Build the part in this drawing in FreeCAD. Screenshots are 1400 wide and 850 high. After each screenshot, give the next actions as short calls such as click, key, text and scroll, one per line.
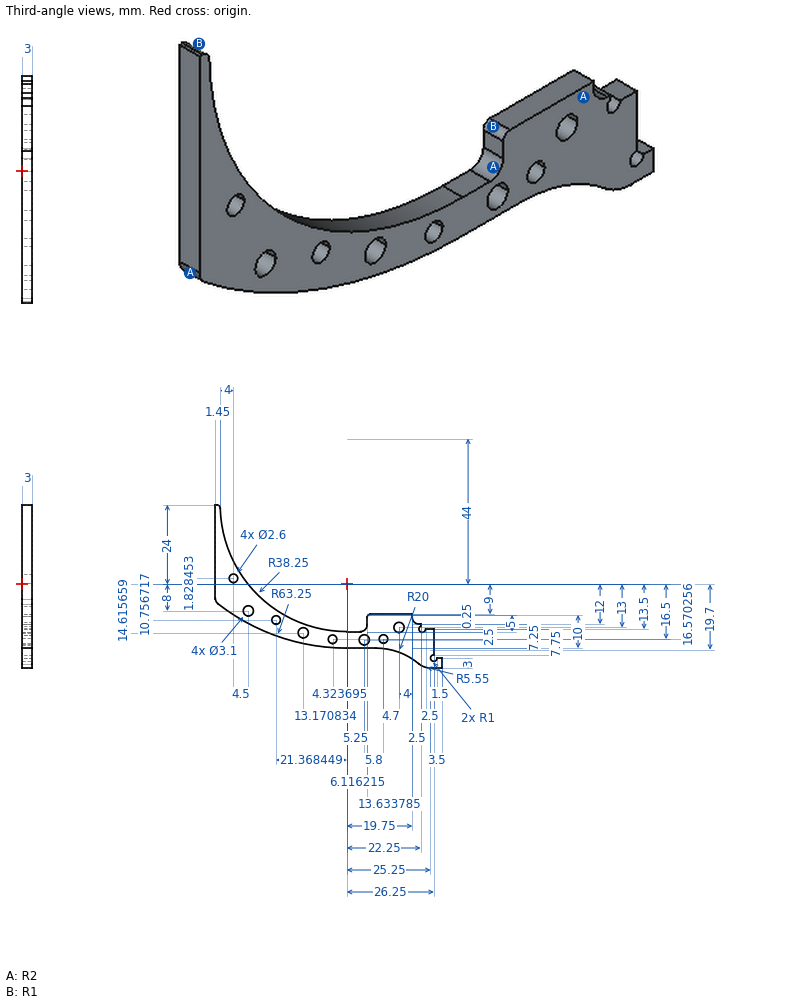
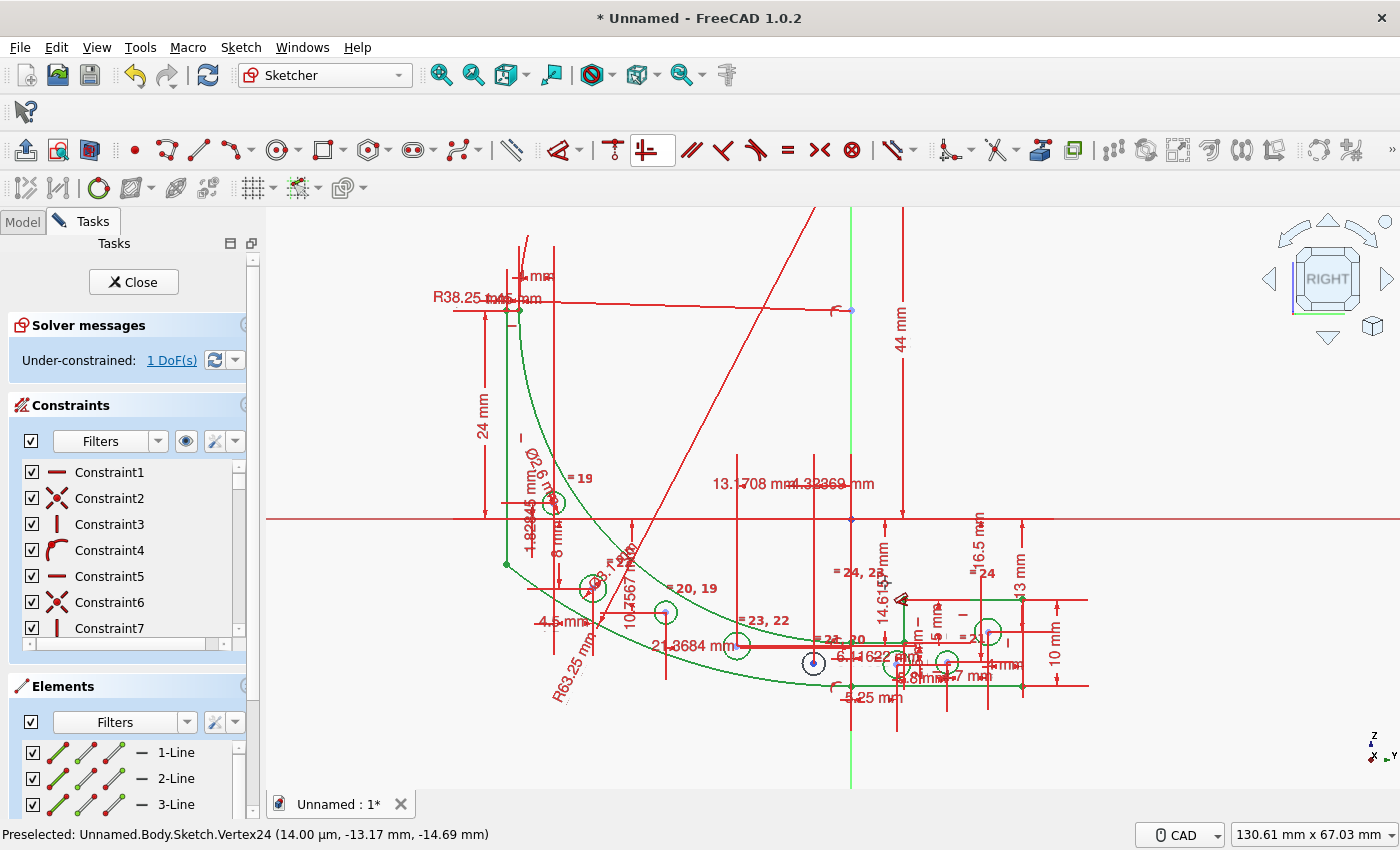
click(814, 664)
click(885, 558)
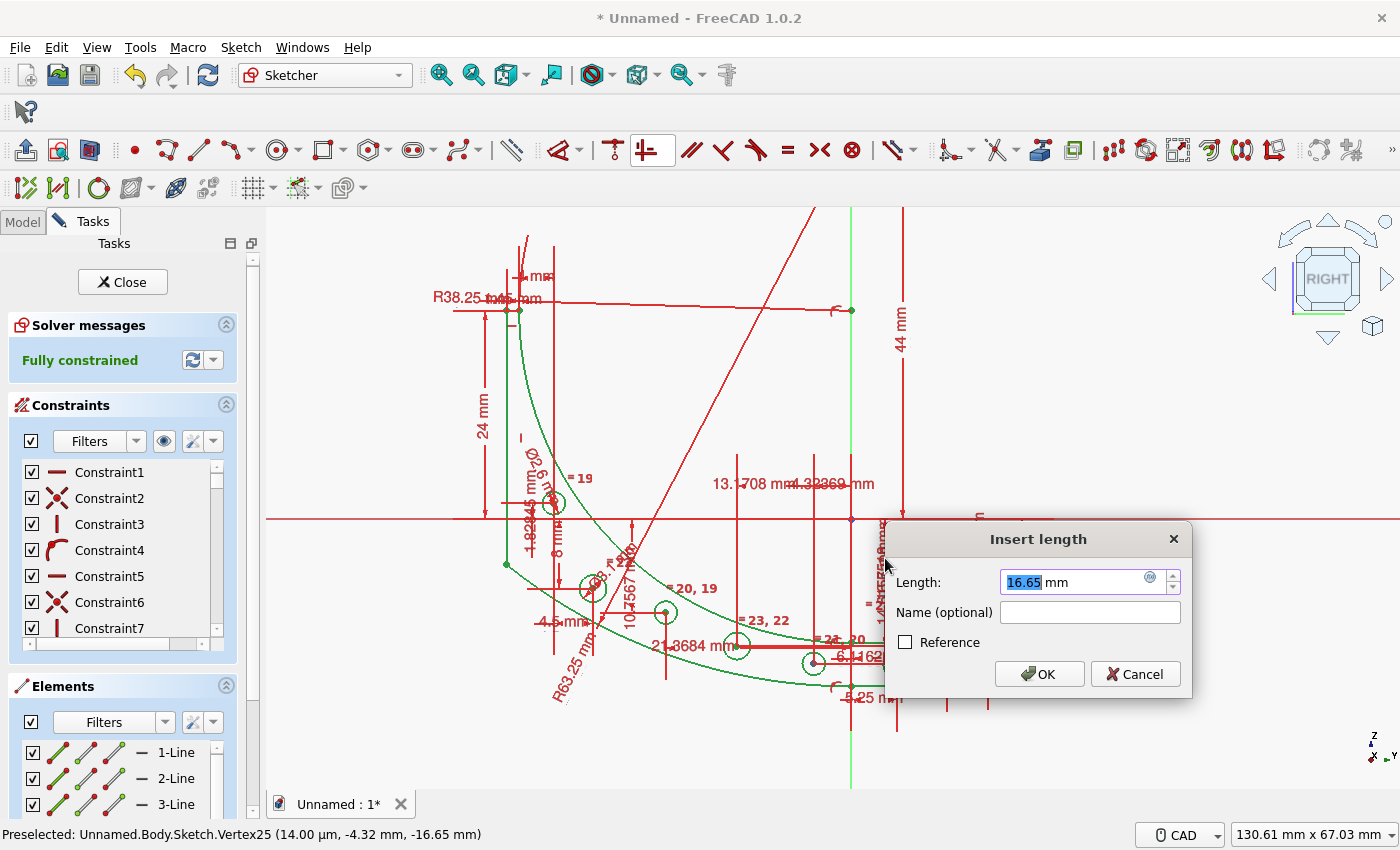
text(16.570256)
key(Return)
key(Escape)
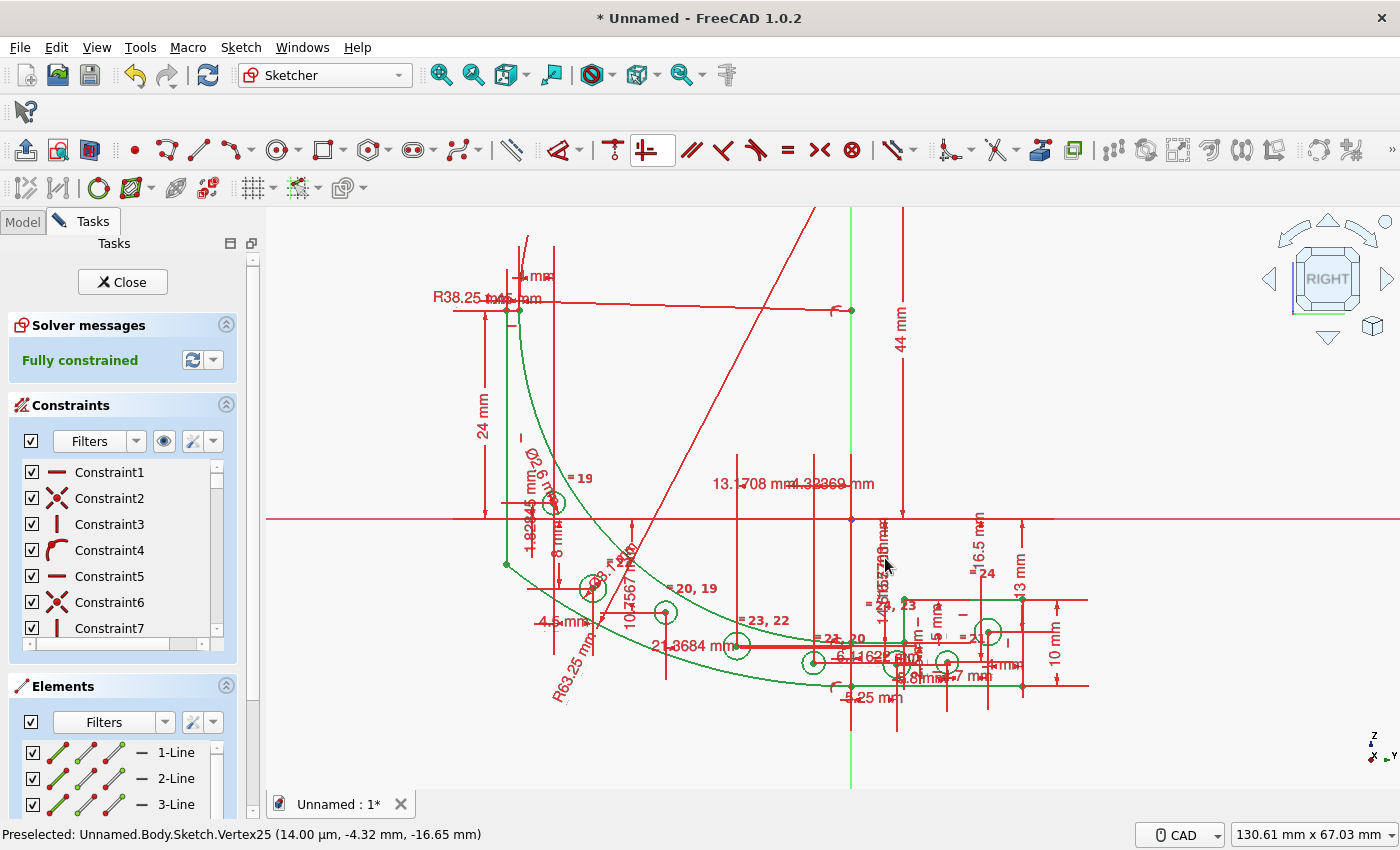
click(123, 282)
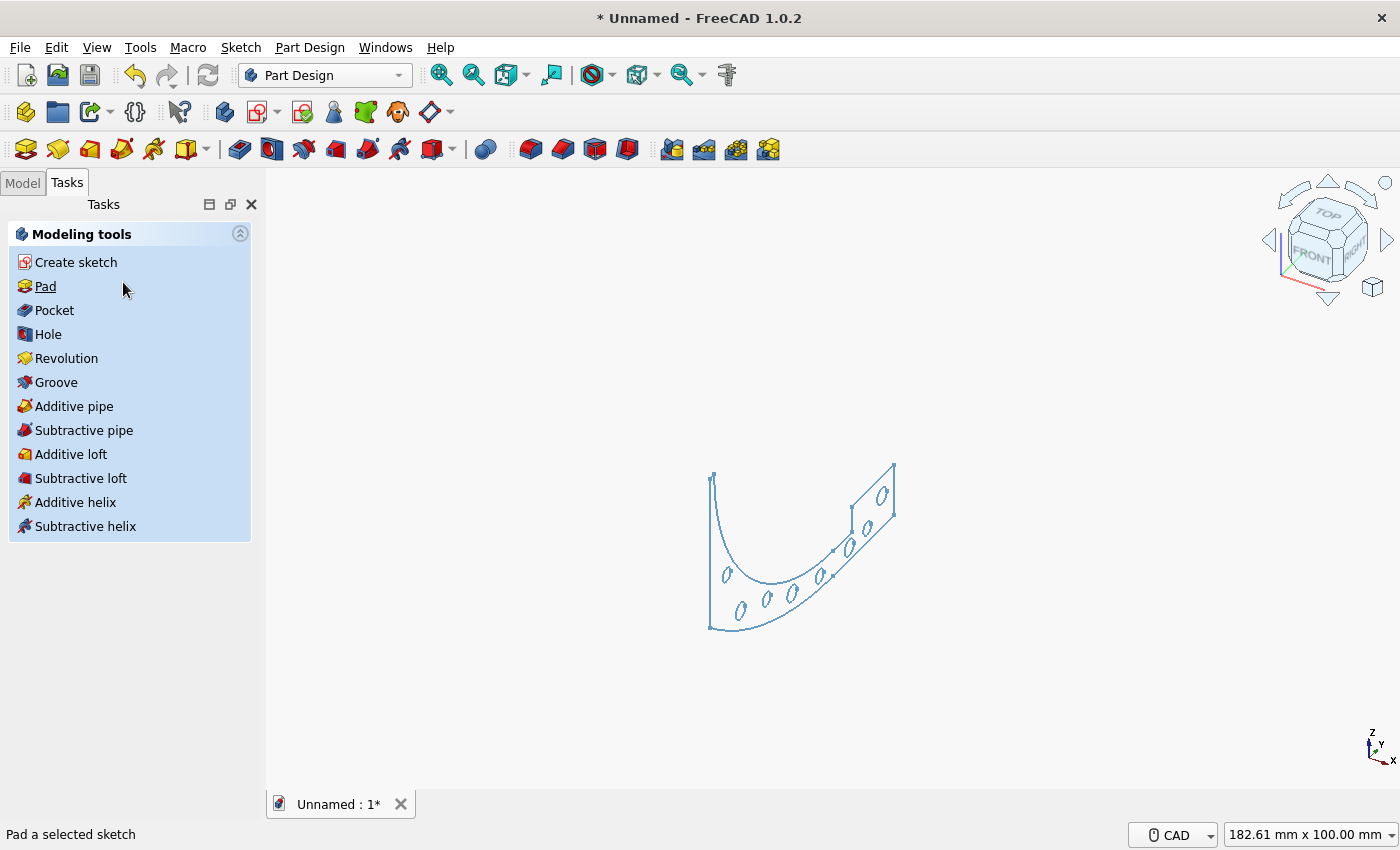
click(26, 150)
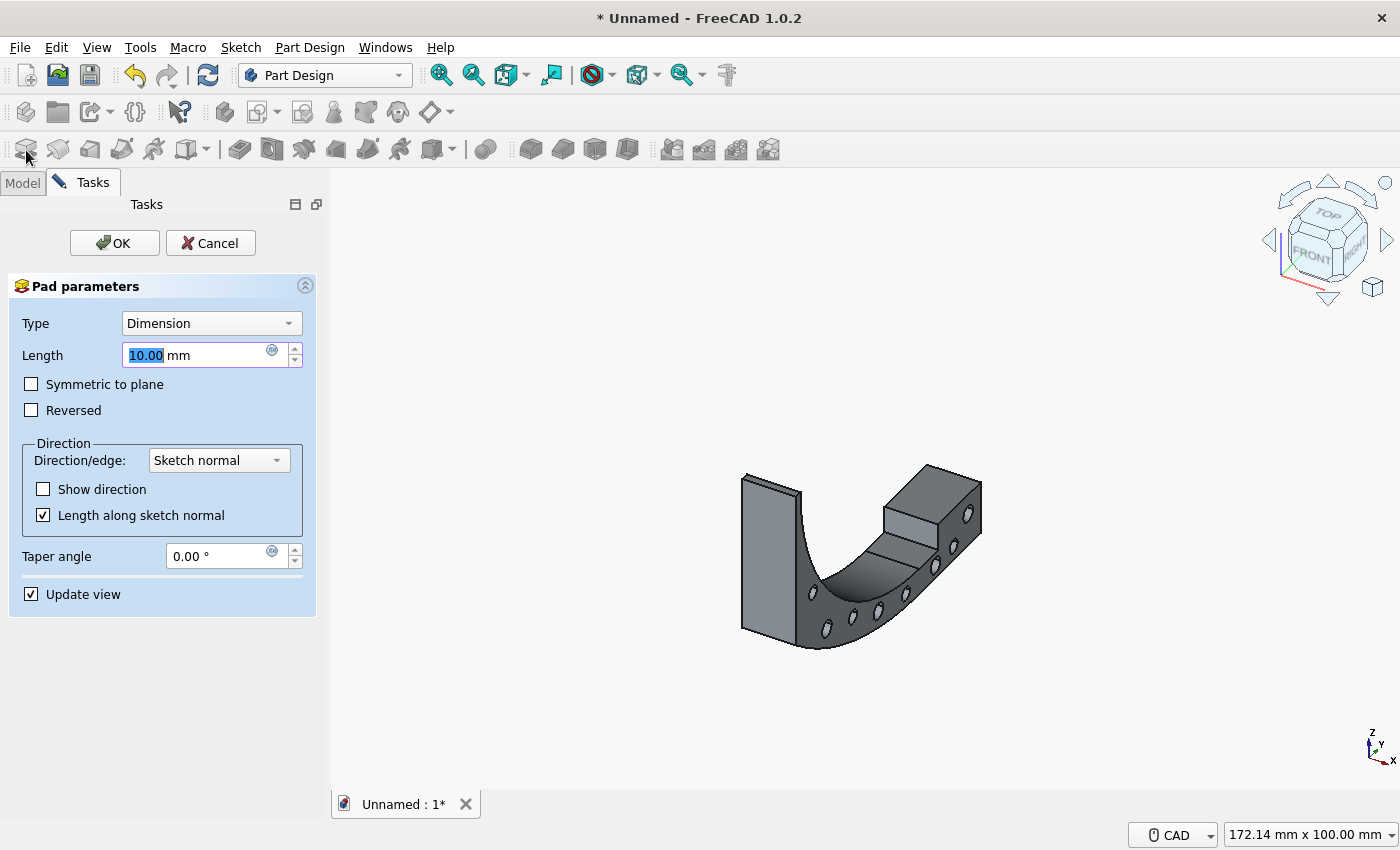
text(3)
key(Tab)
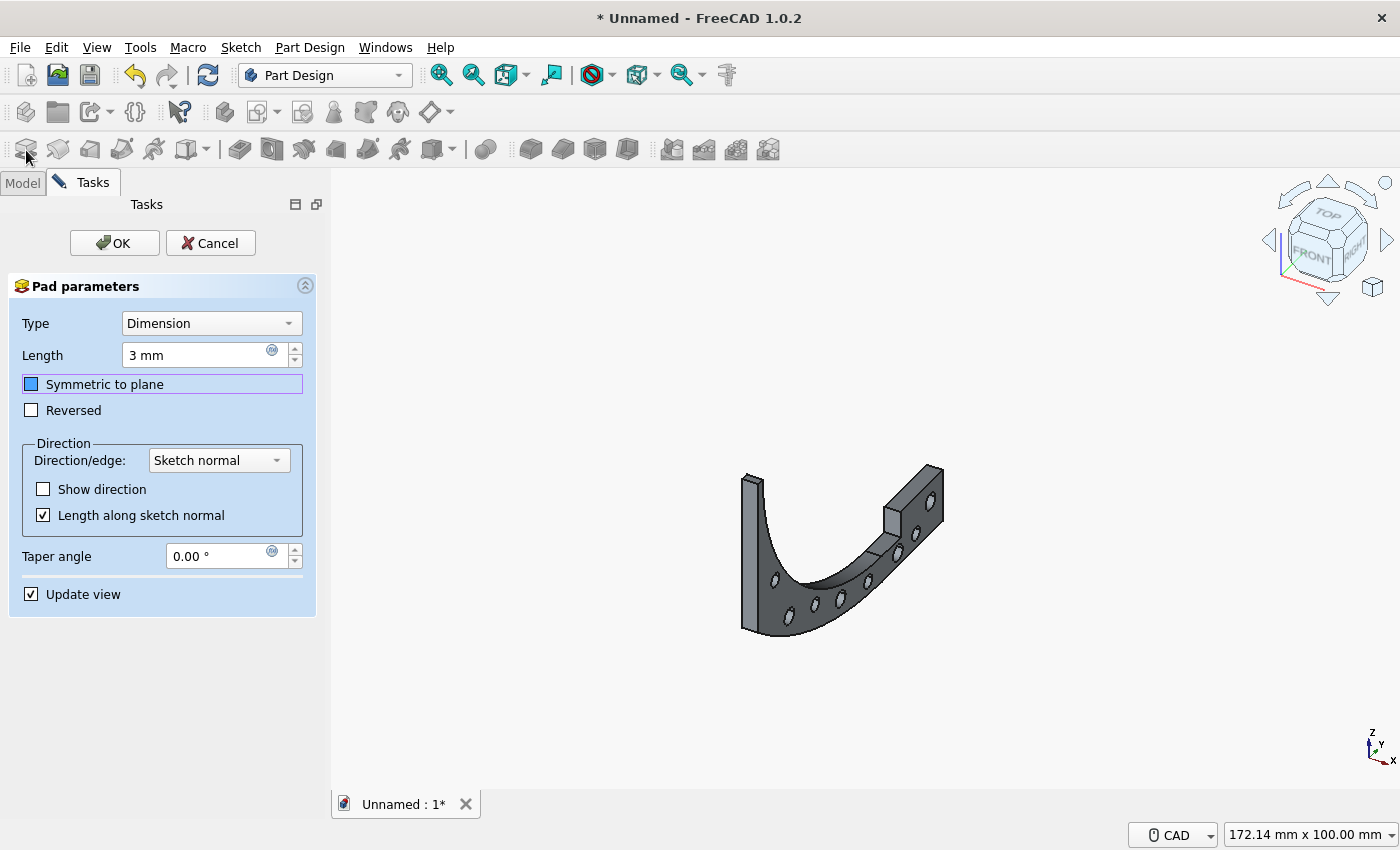
click(115, 243)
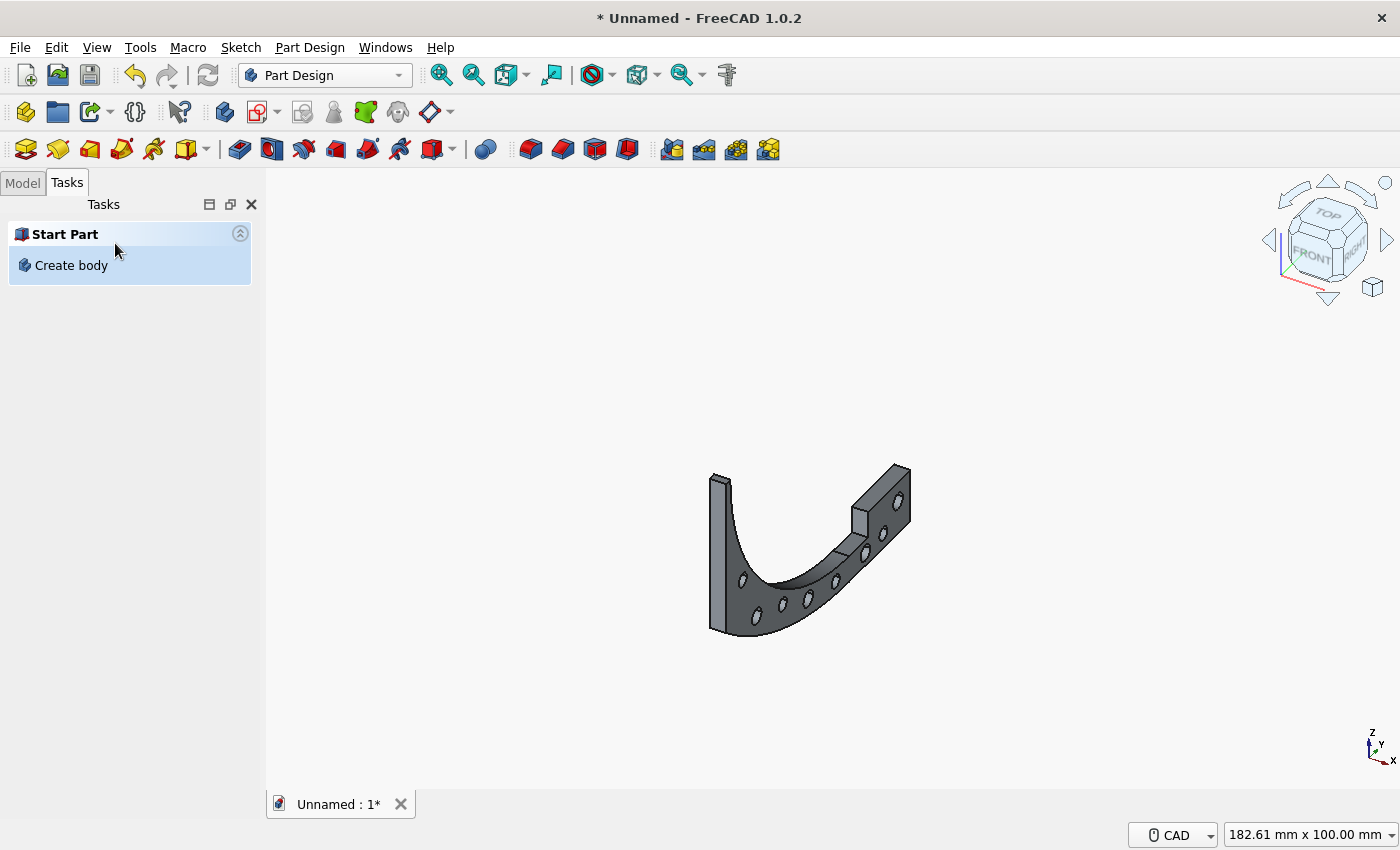
click(739, 612)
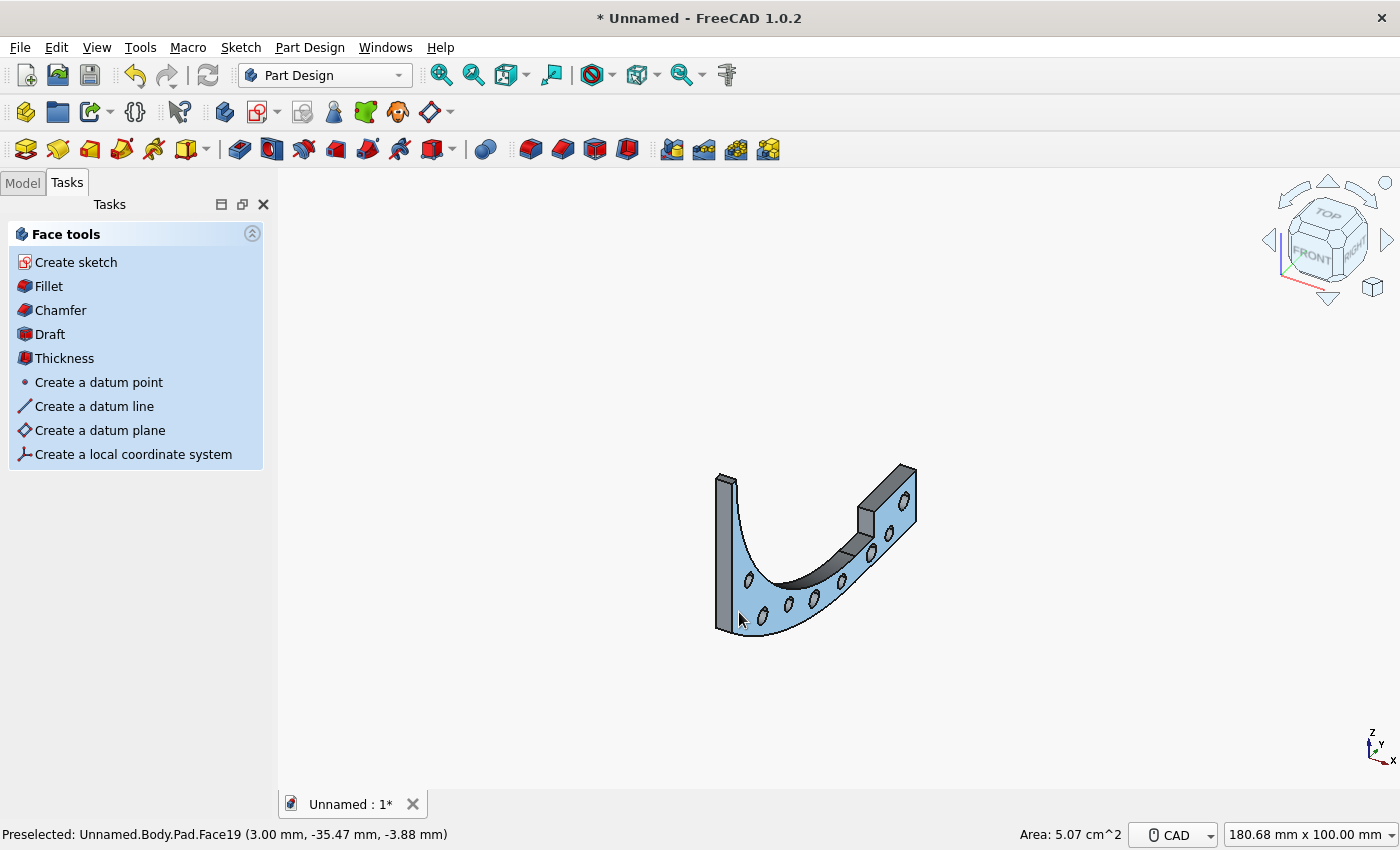
click(258, 112)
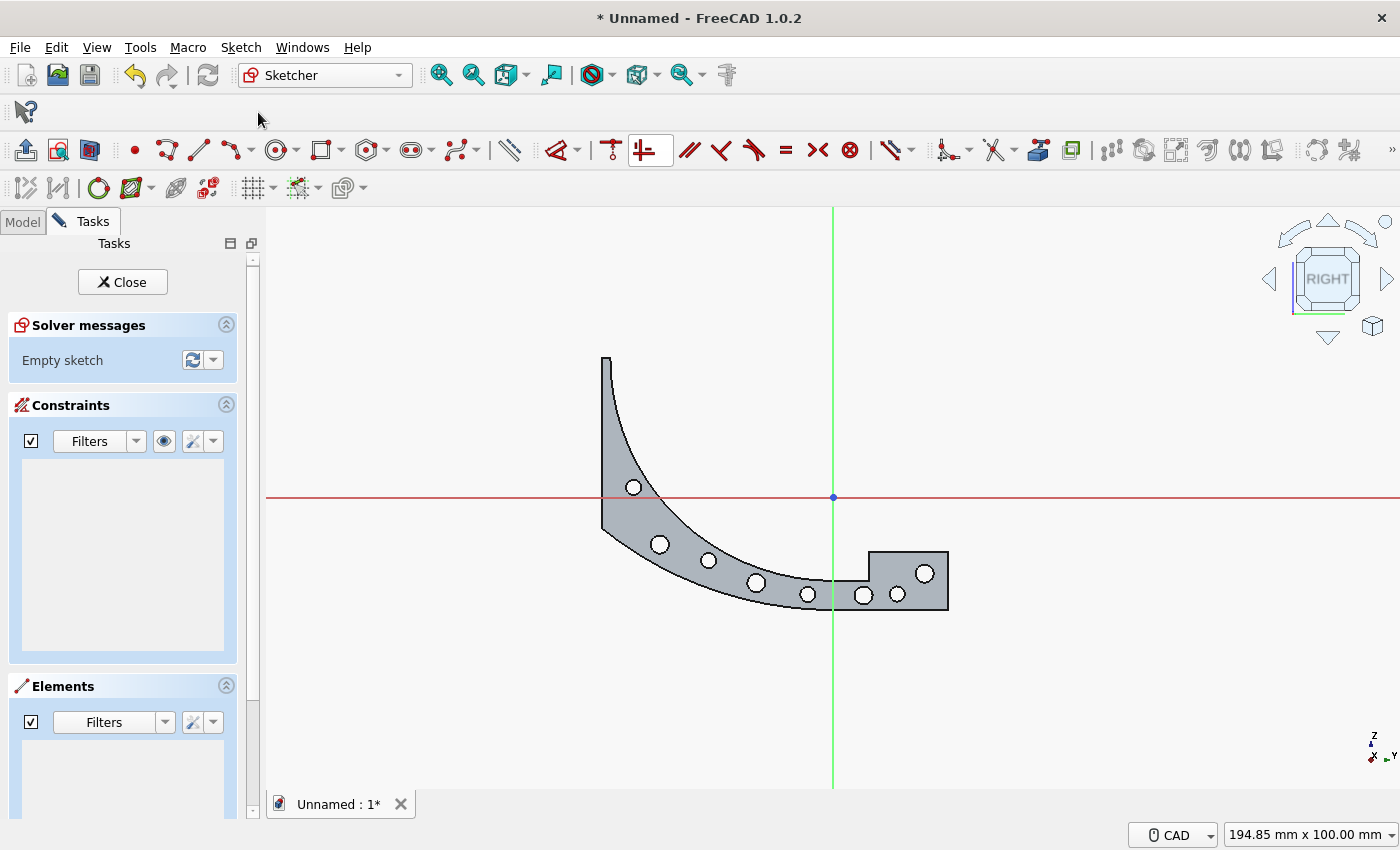
scroll(1005, 614, up, 5)